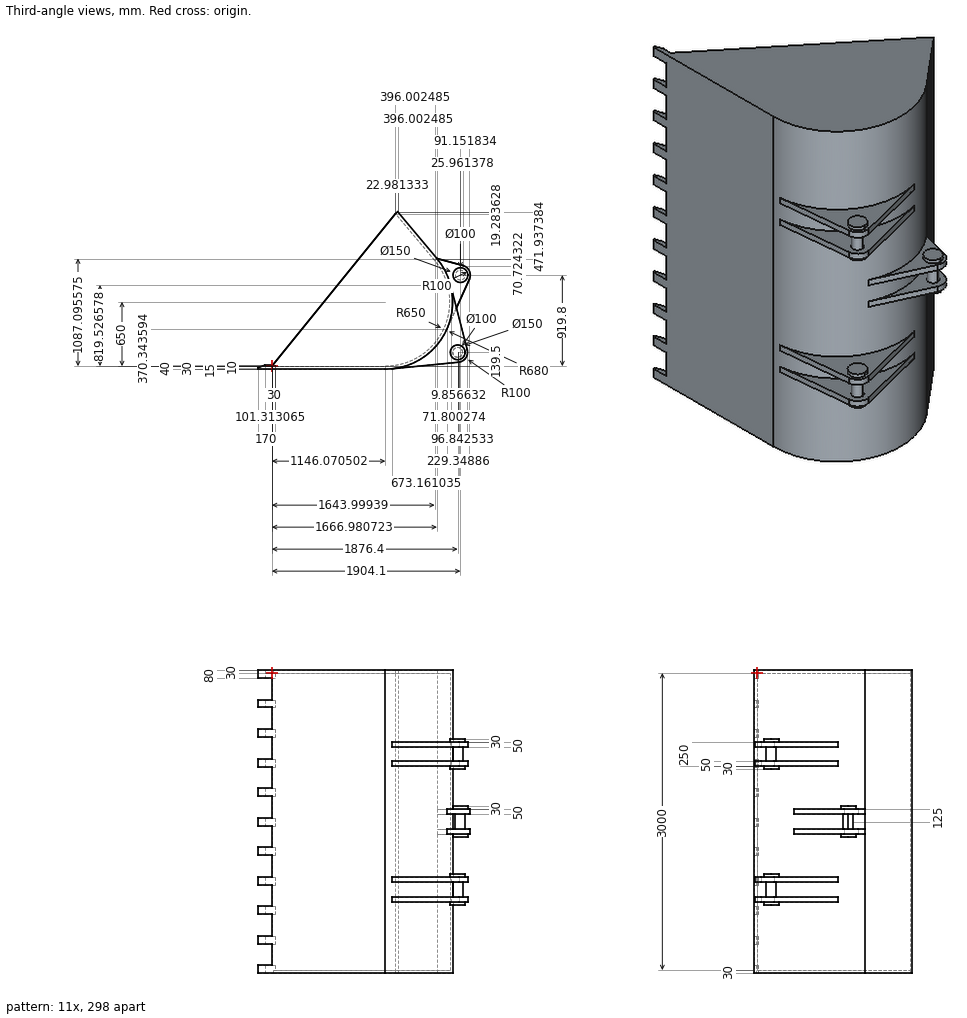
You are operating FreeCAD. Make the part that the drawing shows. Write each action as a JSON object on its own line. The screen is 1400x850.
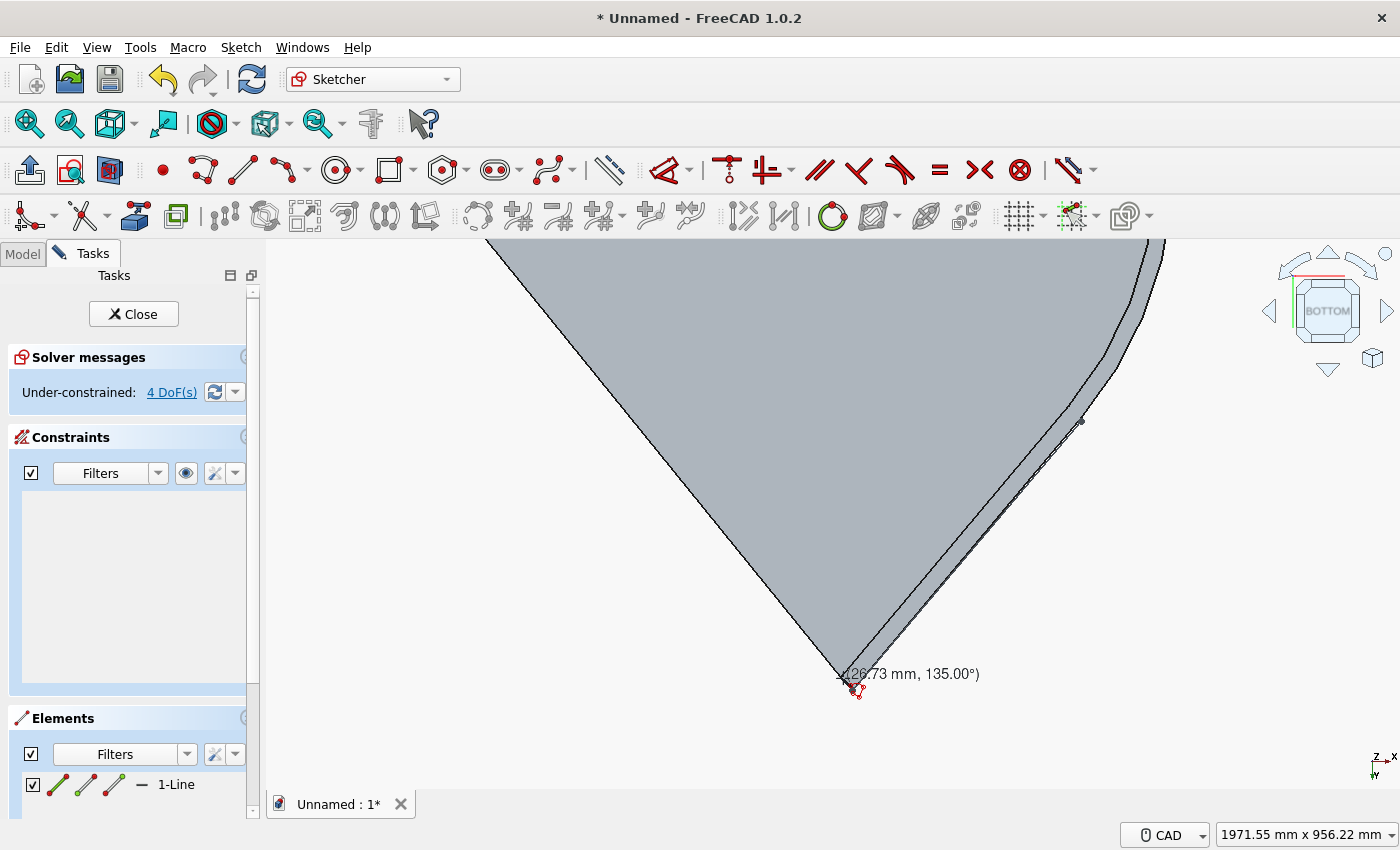
{"action": "left_click", "coordinate": [841, 677]}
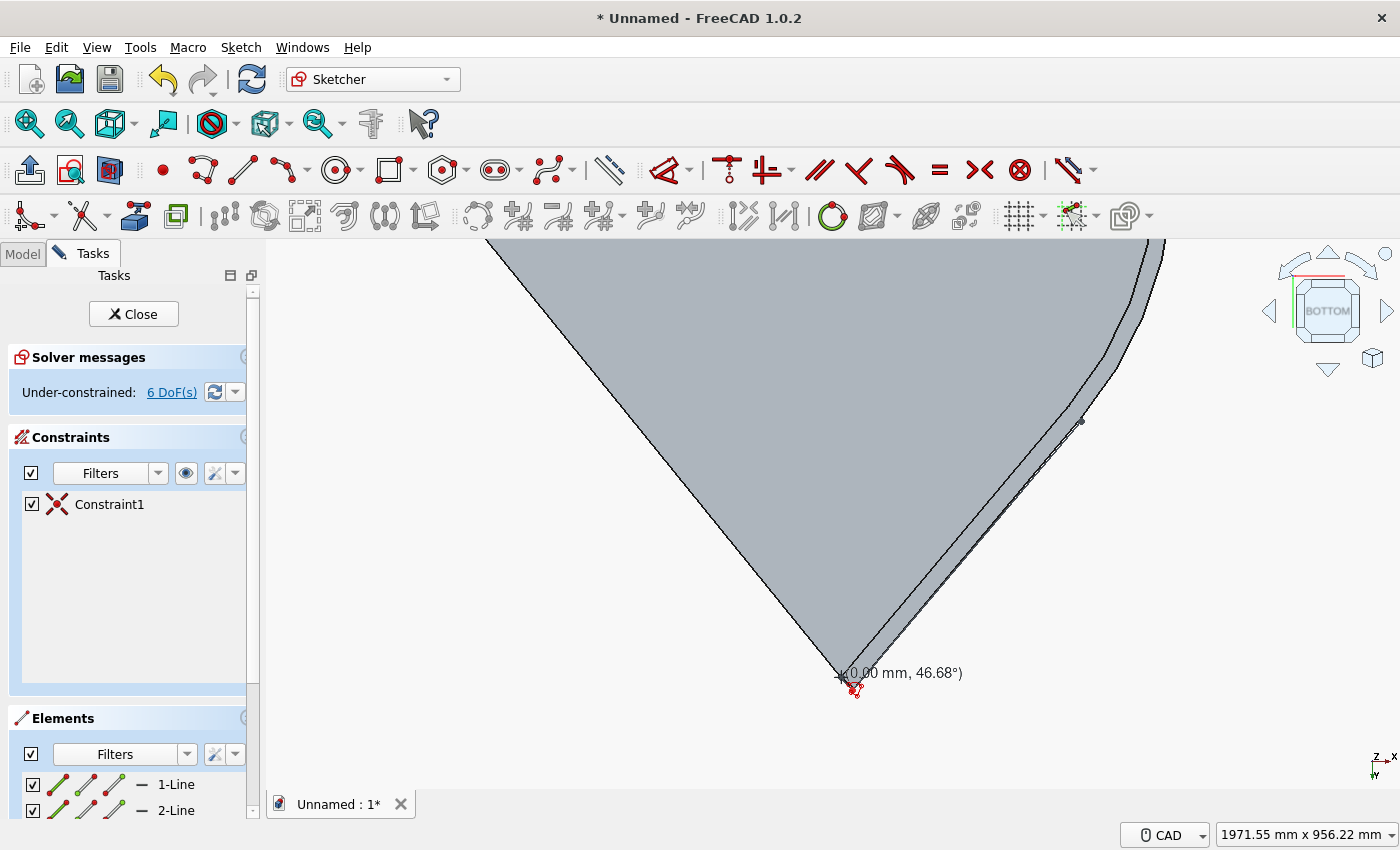
{"action": "scroll", "coordinate": [843, 678], "scroll_direction": "down", "scroll_amount": 5}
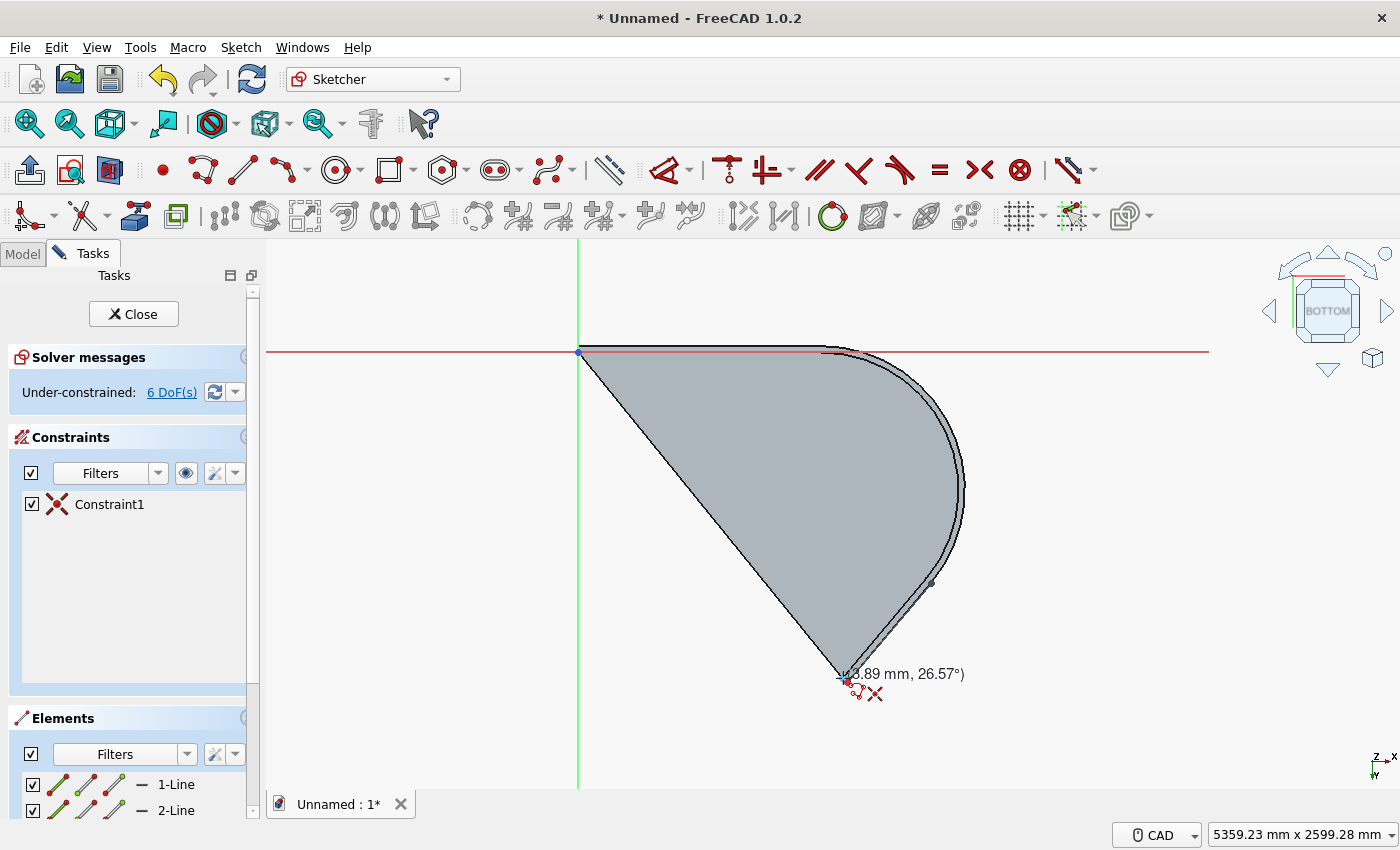
{"action": "left_click", "coordinate": [578, 352]}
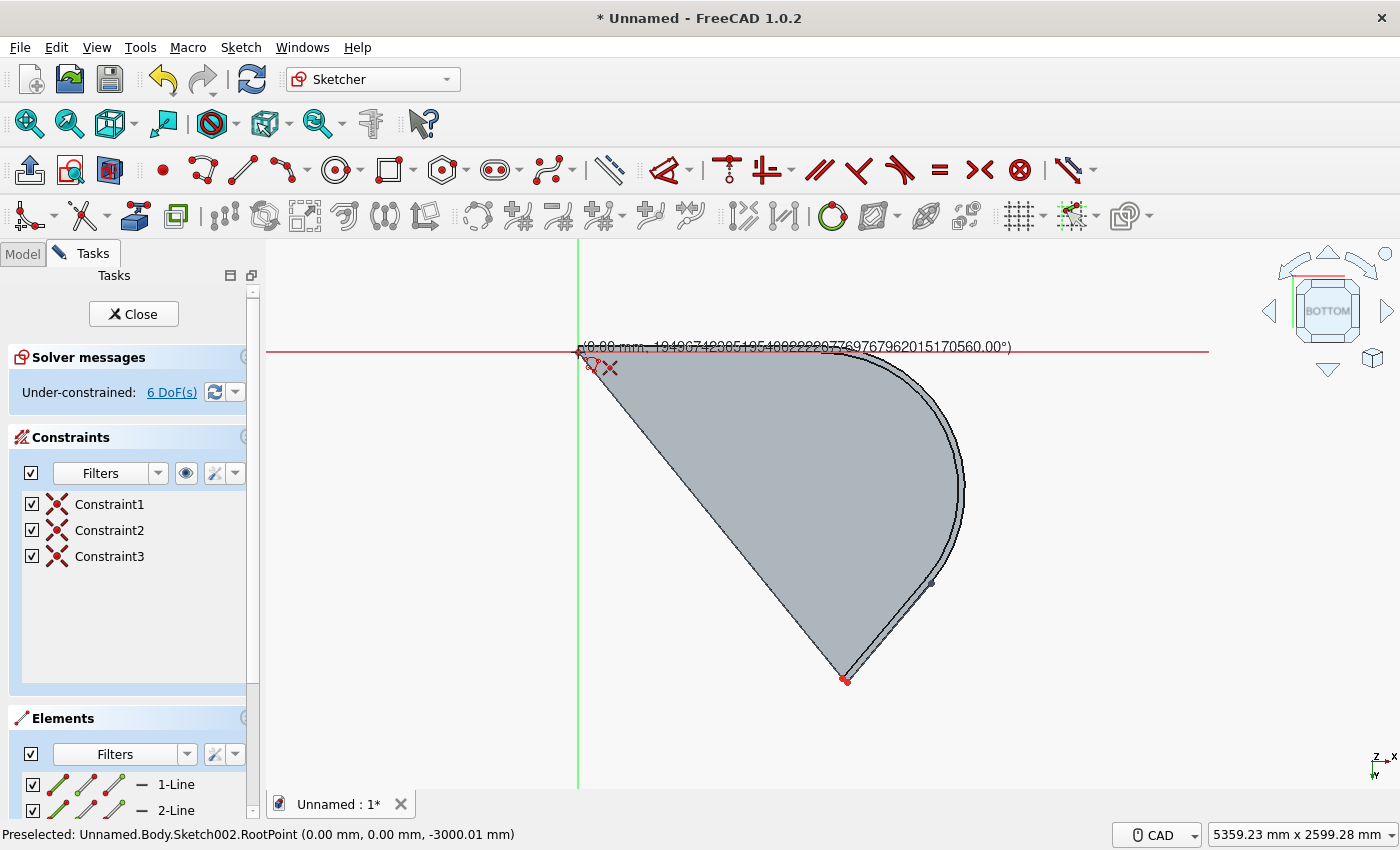
{"action": "scroll", "coordinate": [578, 346], "scroll_direction": "up", "scroll_amount": 5}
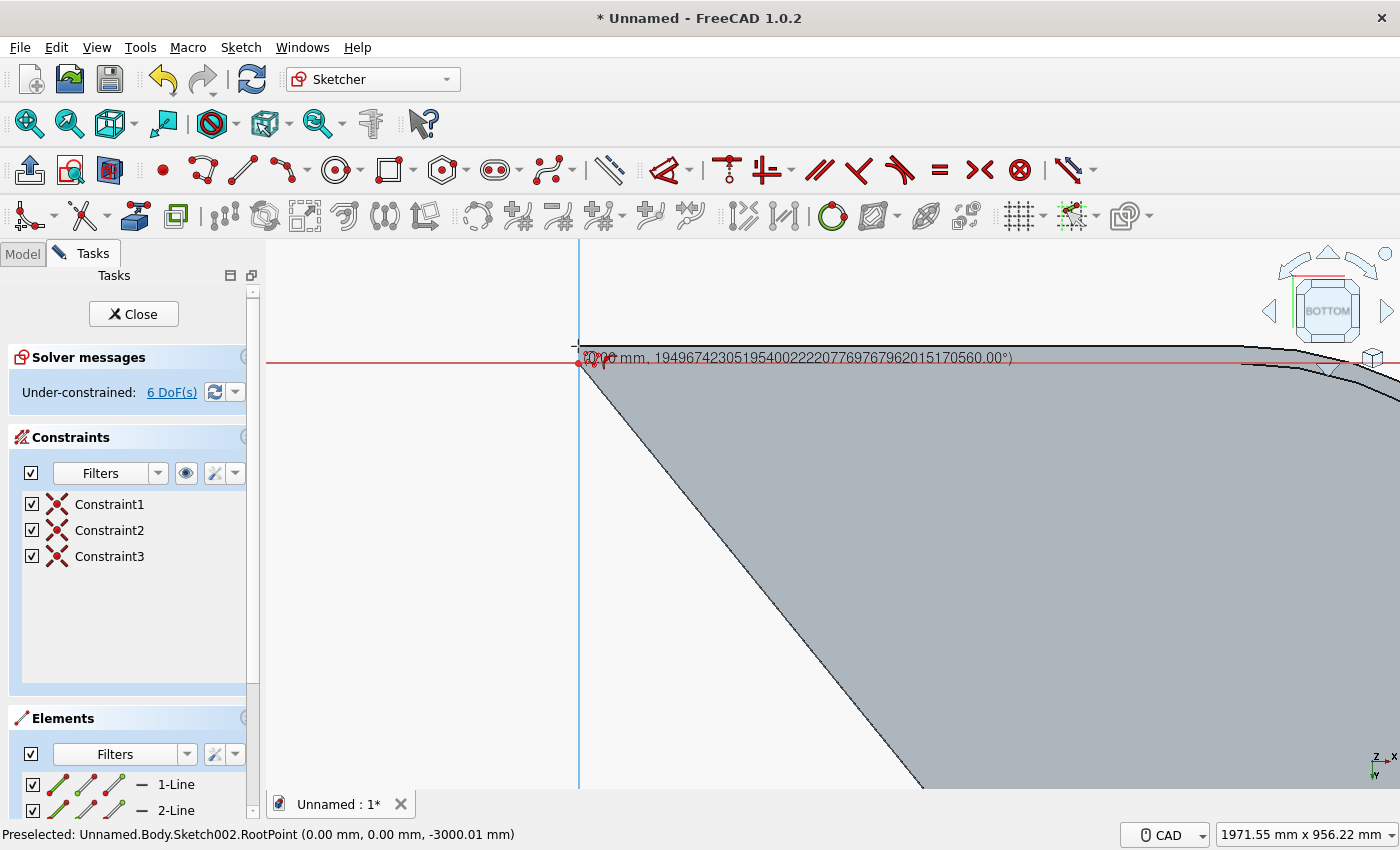
{"action": "left_click", "coordinate": [588, 346]}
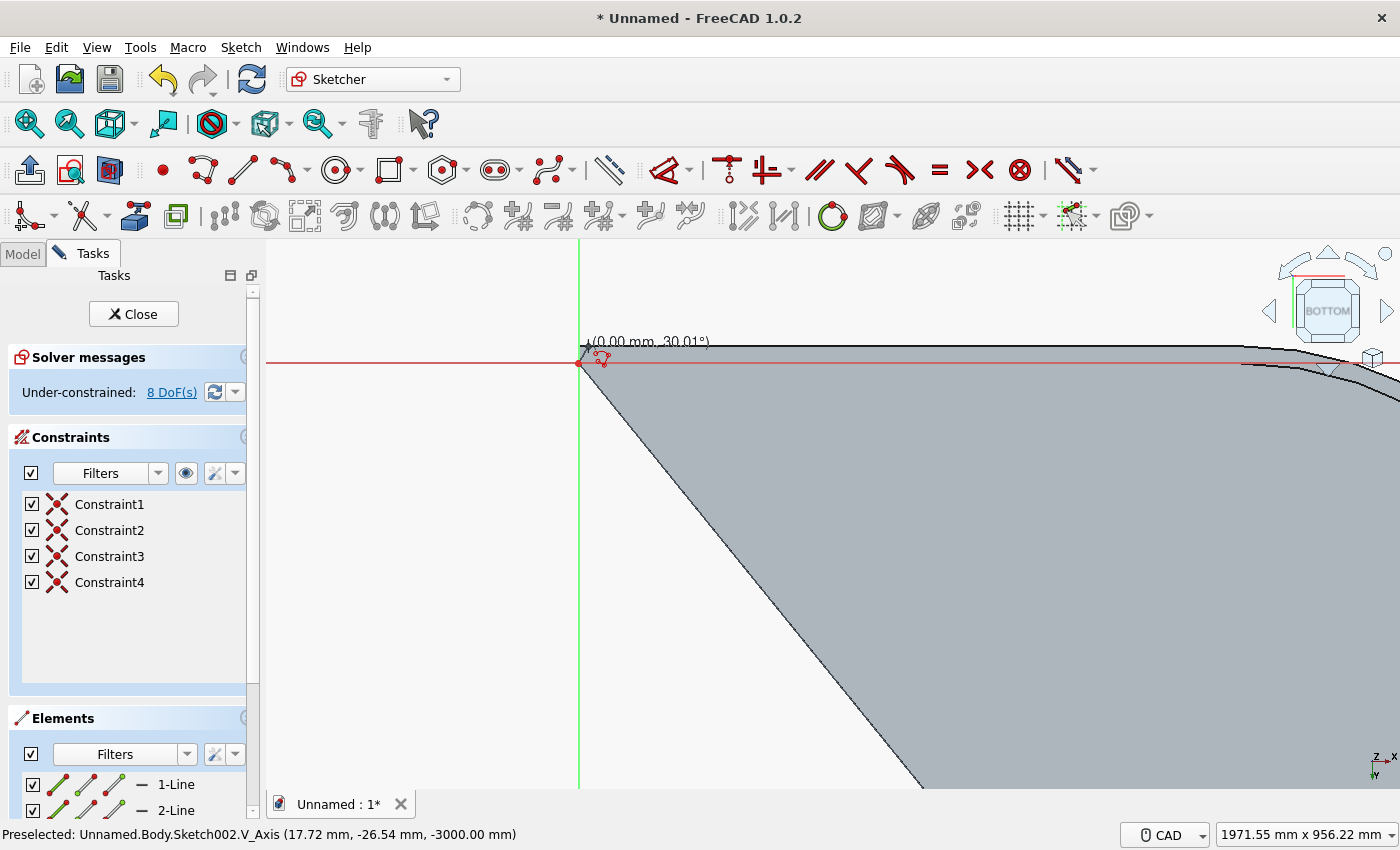
{"action": "scroll", "coordinate": [578, 346], "scroll_direction": "down", "scroll_amount": 5}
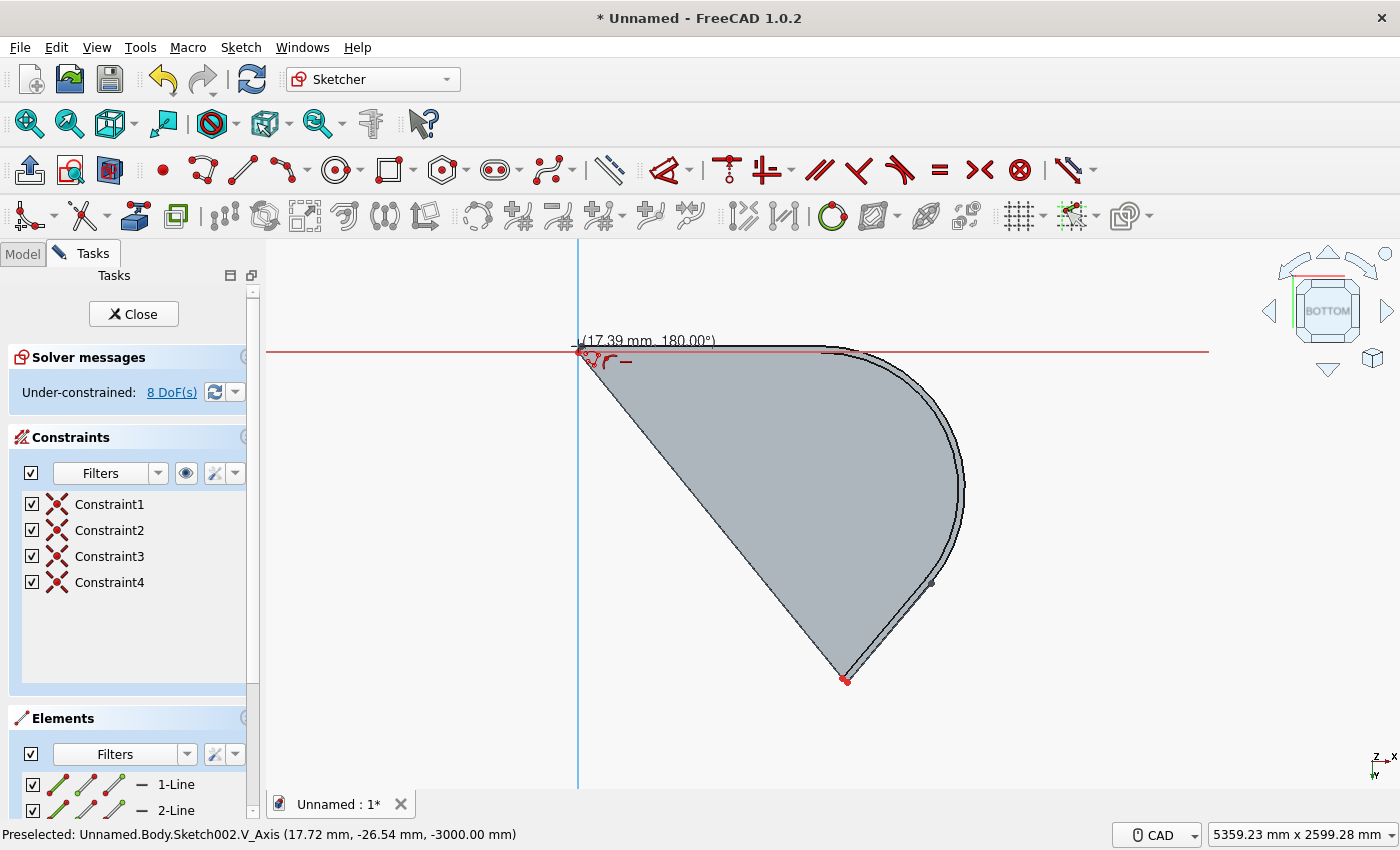
{"action": "scroll", "coordinate": [821, 346], "scroll_direction": "up", "scroll_amount": 5}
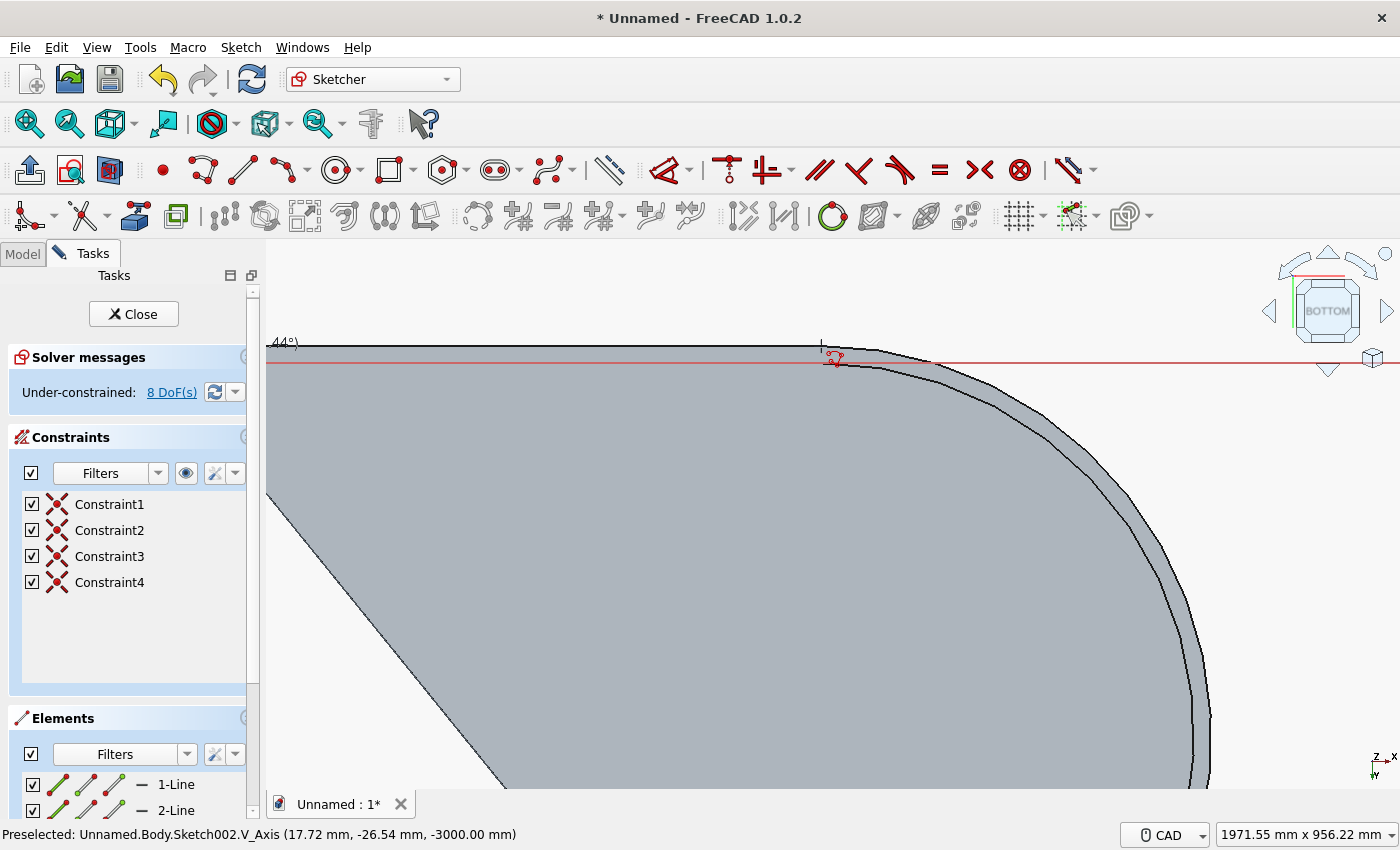
{"action": "left_click", "coordinate": [820, 346]}
{"action": "right_click", "coordinate": [820, 346]}